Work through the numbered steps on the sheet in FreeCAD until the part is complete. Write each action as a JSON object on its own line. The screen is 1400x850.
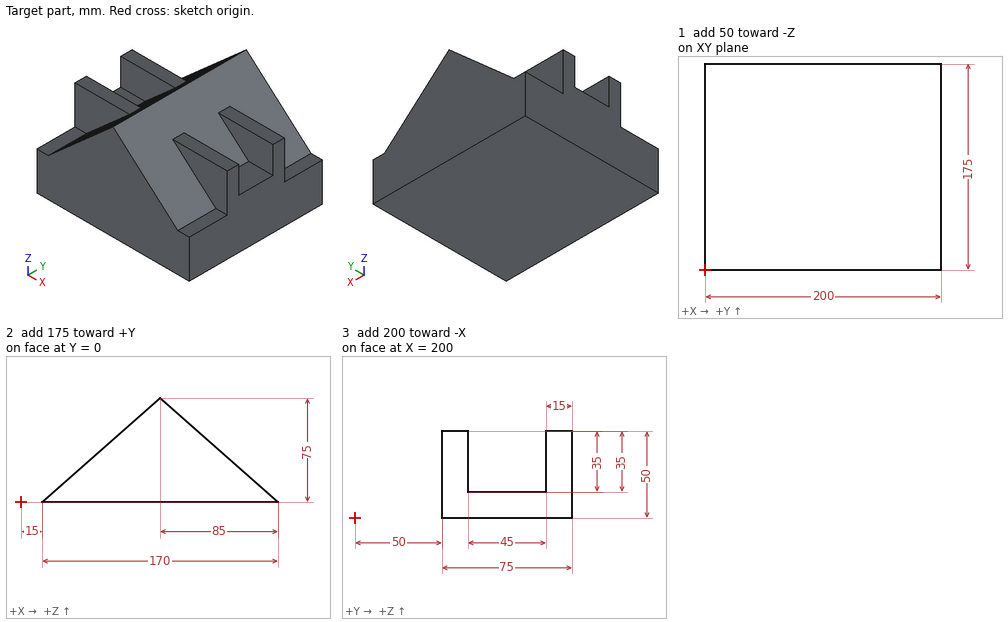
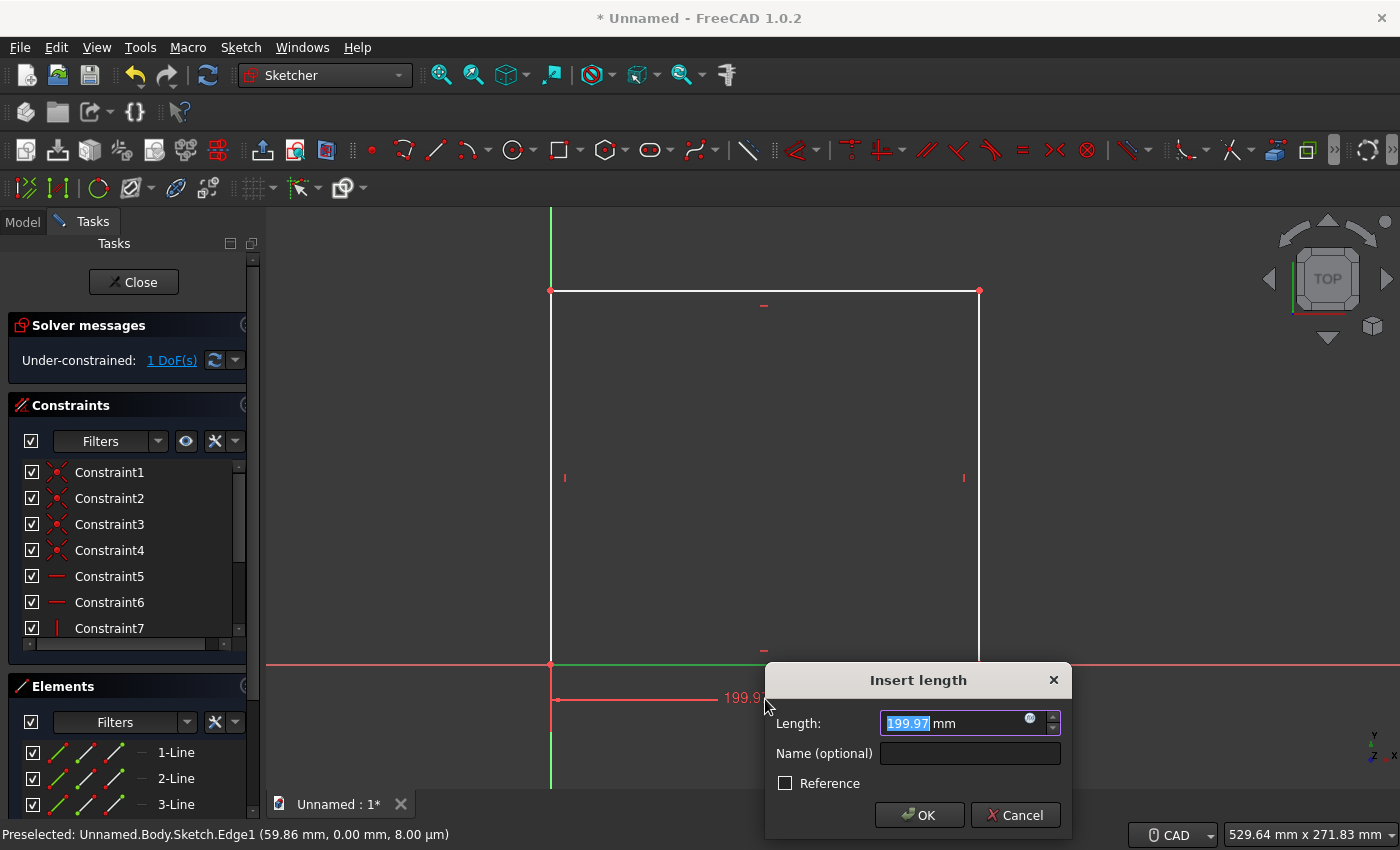
{"action": "type", "text": "200"}
{"action": "key", "text": "Return"}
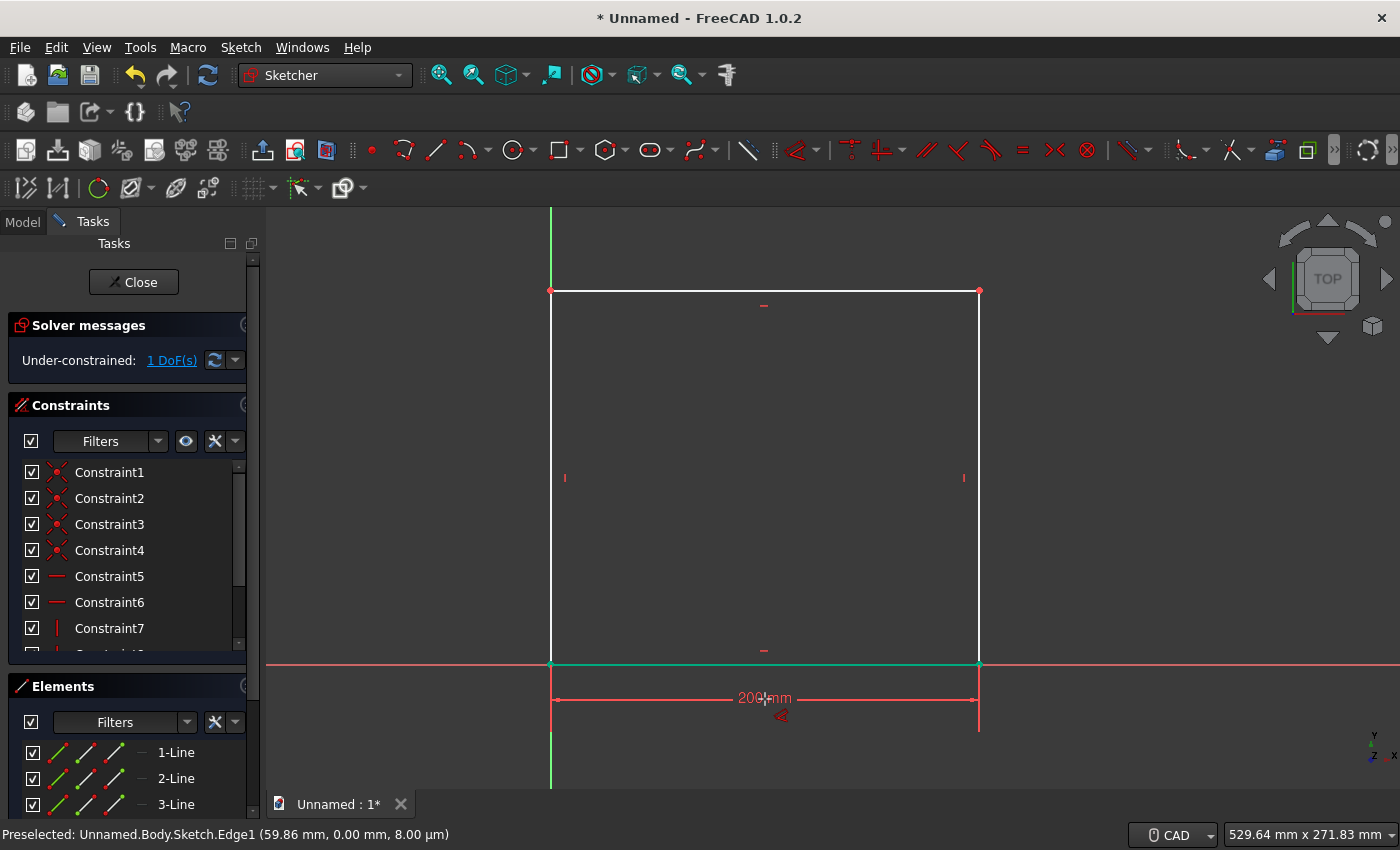
{"action": "left_click", "coordinate": [979, 553]}
{"action": "left_click", "coordinate": [1013, 478]}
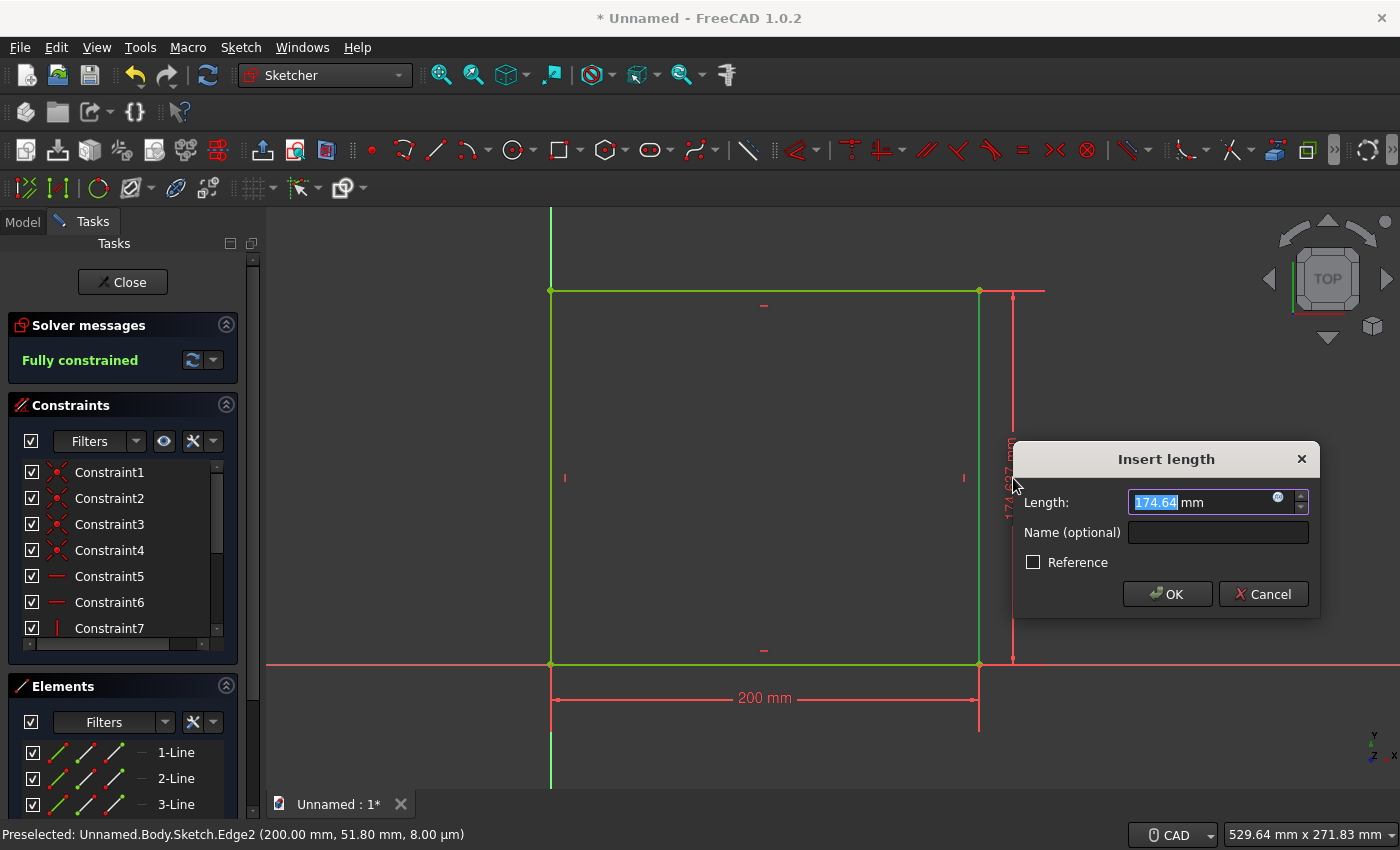
{"action": "type", "text": "175"}
{"action": "key", "text": "Return"}
{"action": "key", "text": "Escape"}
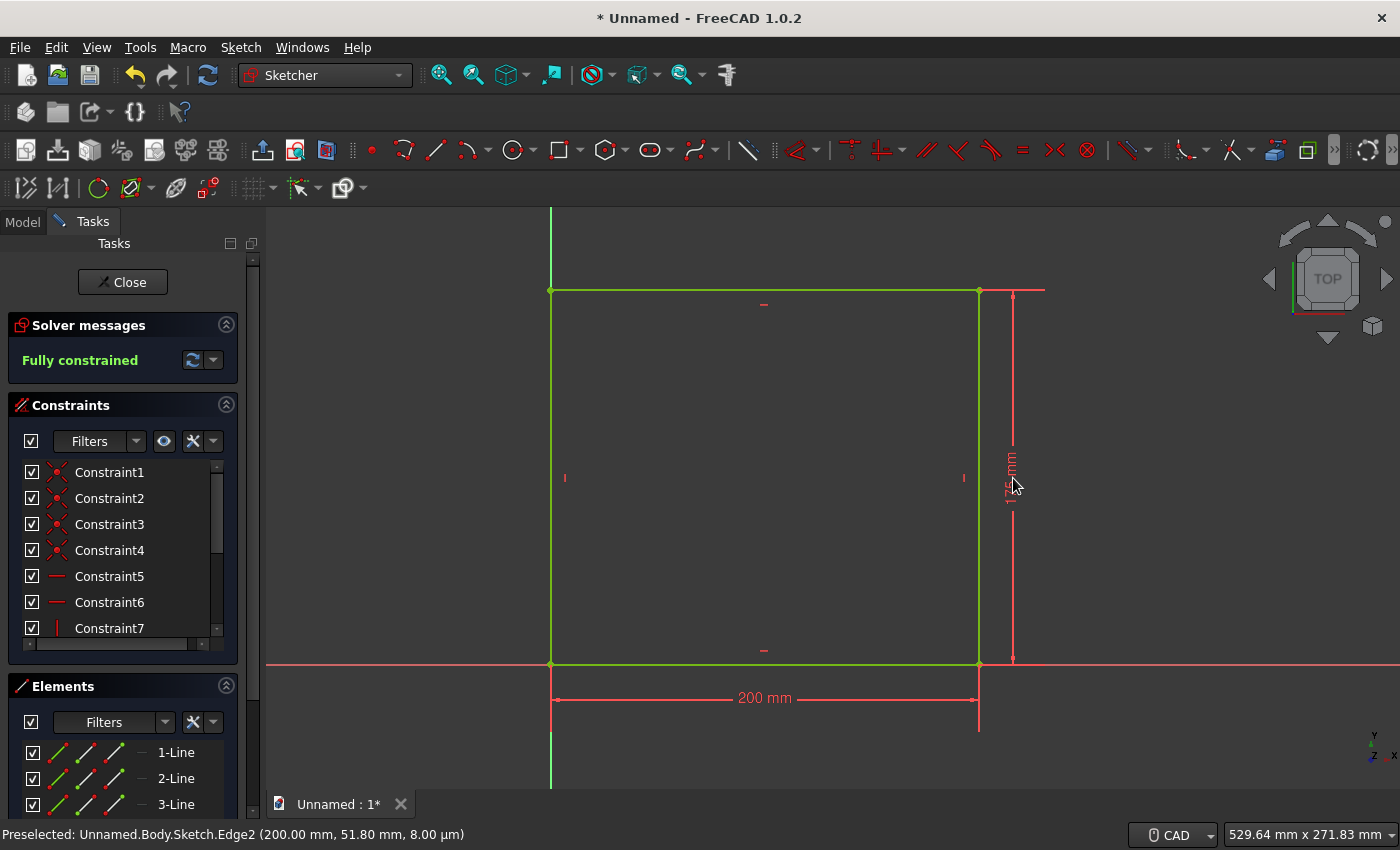
{"action": "left_click", "coordinate": [123, 282]}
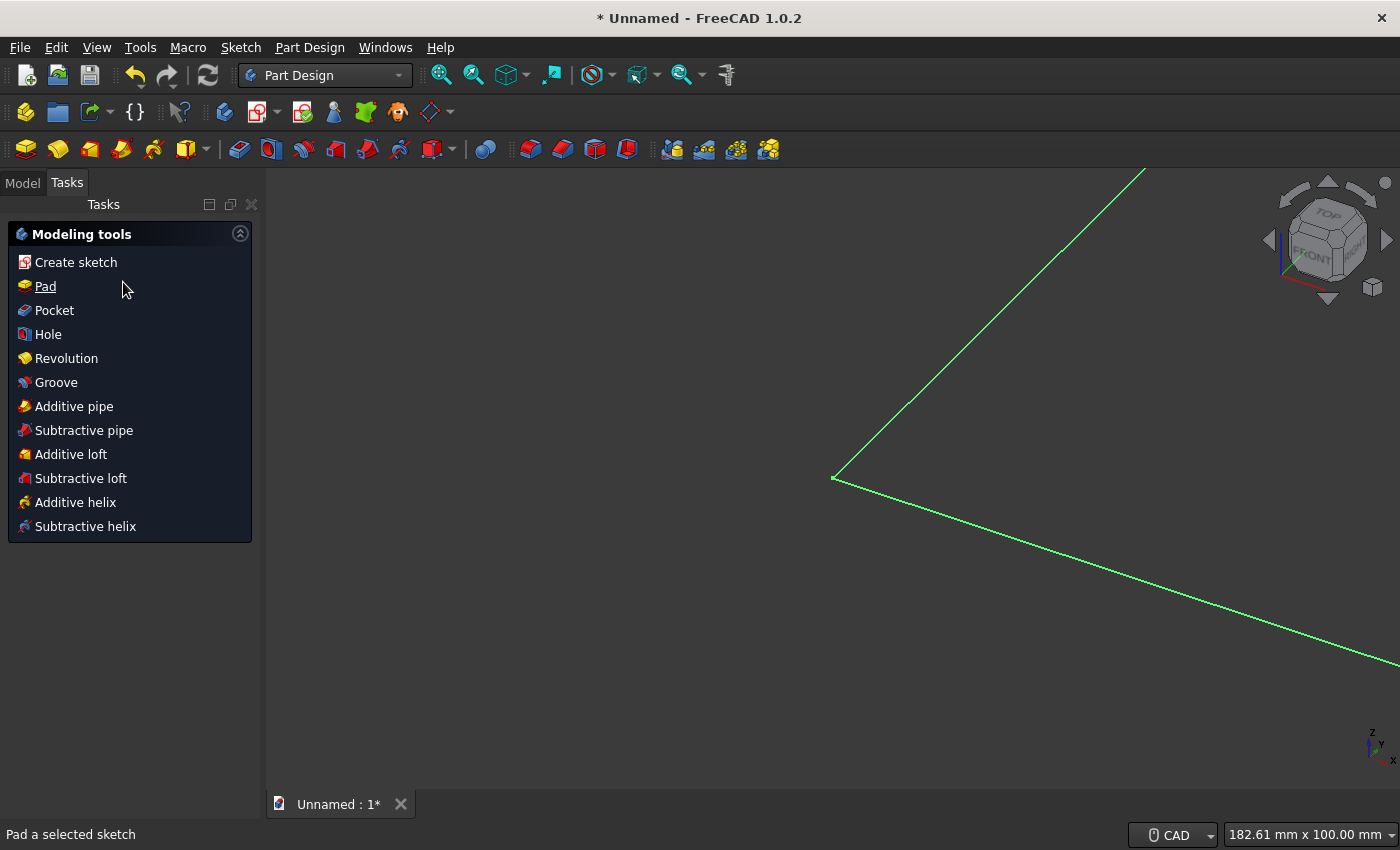
{"action": "left_click", "coordinate": [26, 150]}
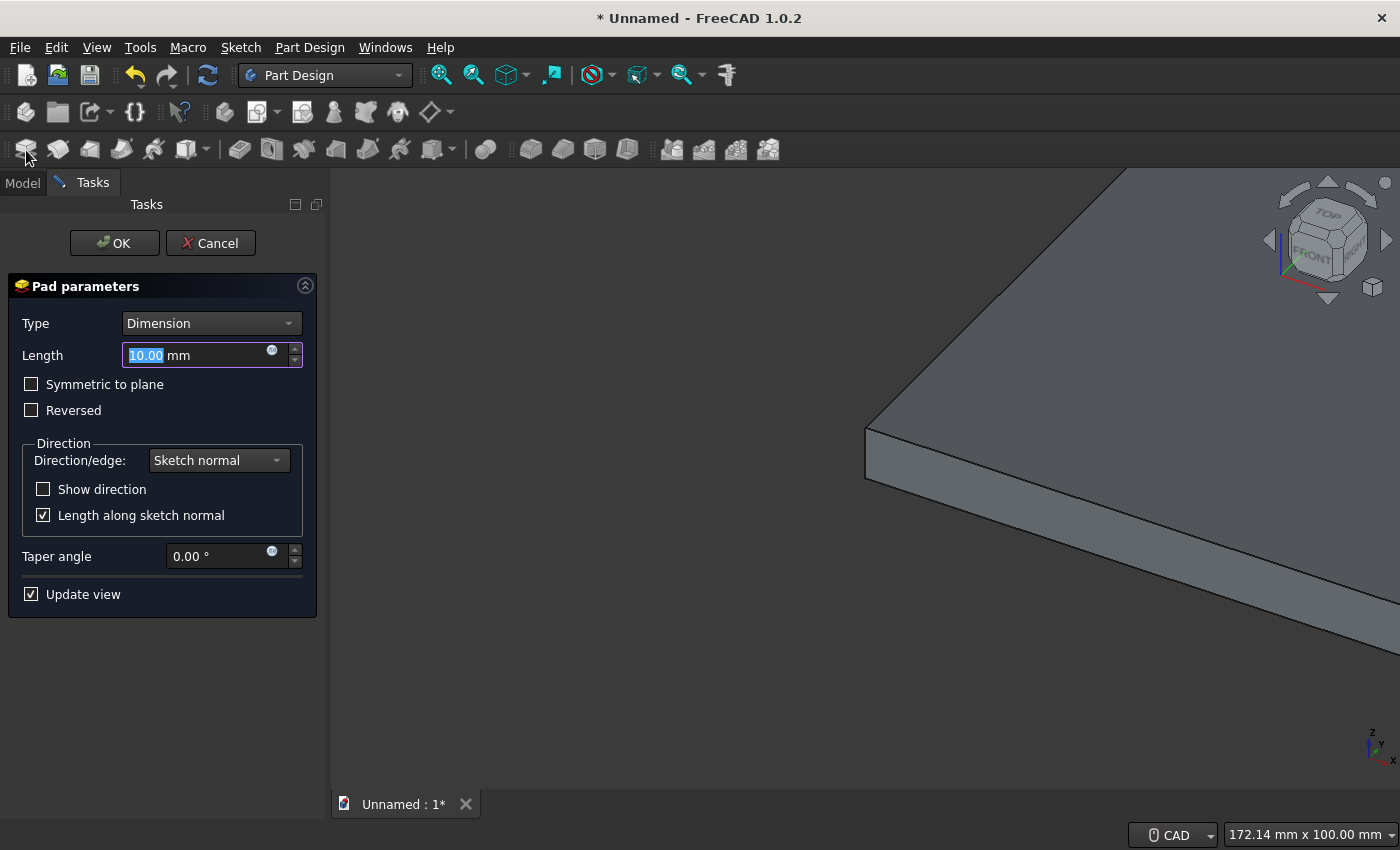
{"action": "type", "text": "50"}
{"action": "key", "text": "Tab"}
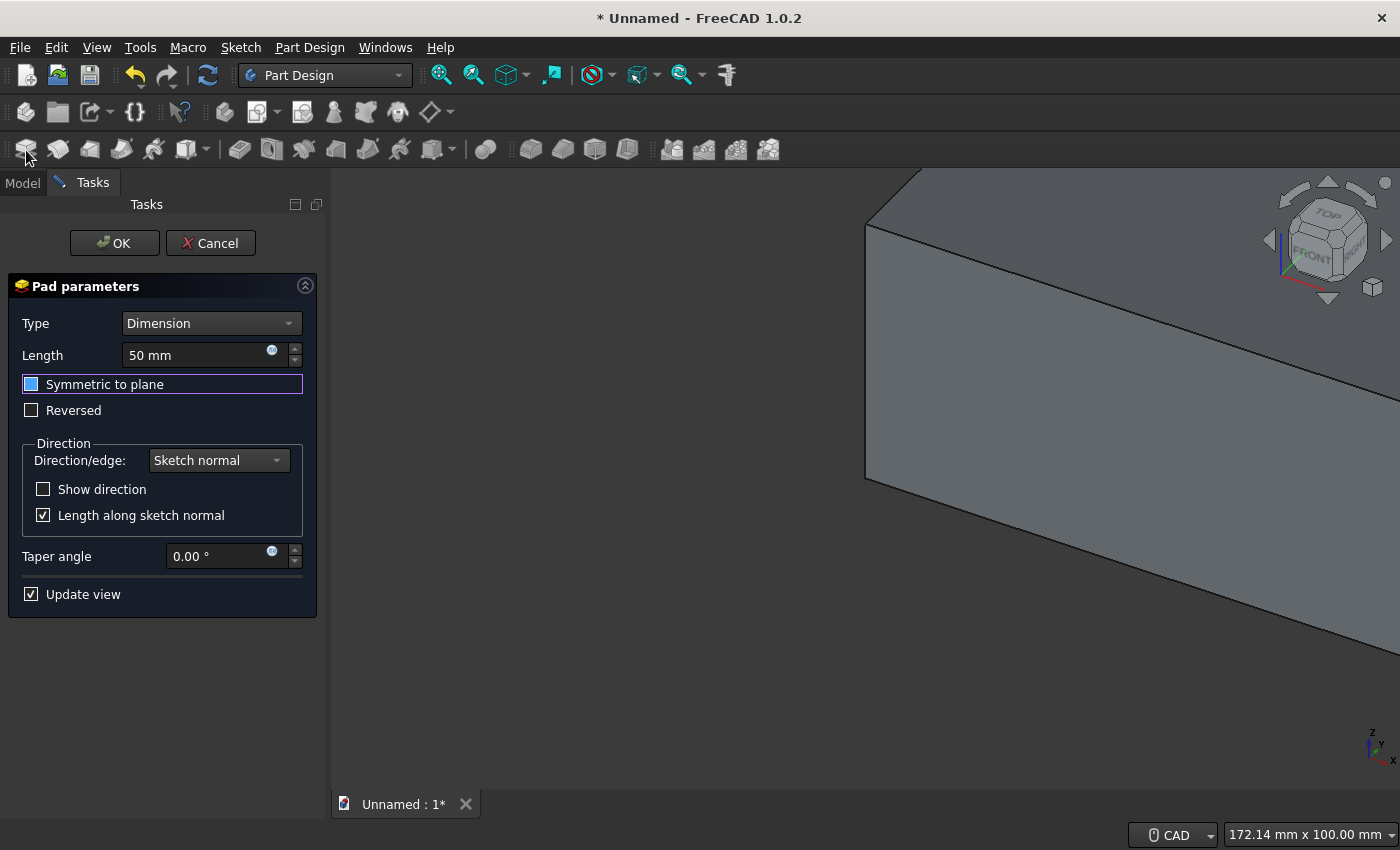
{"action": "left_click", "coordinate": [30, 410]}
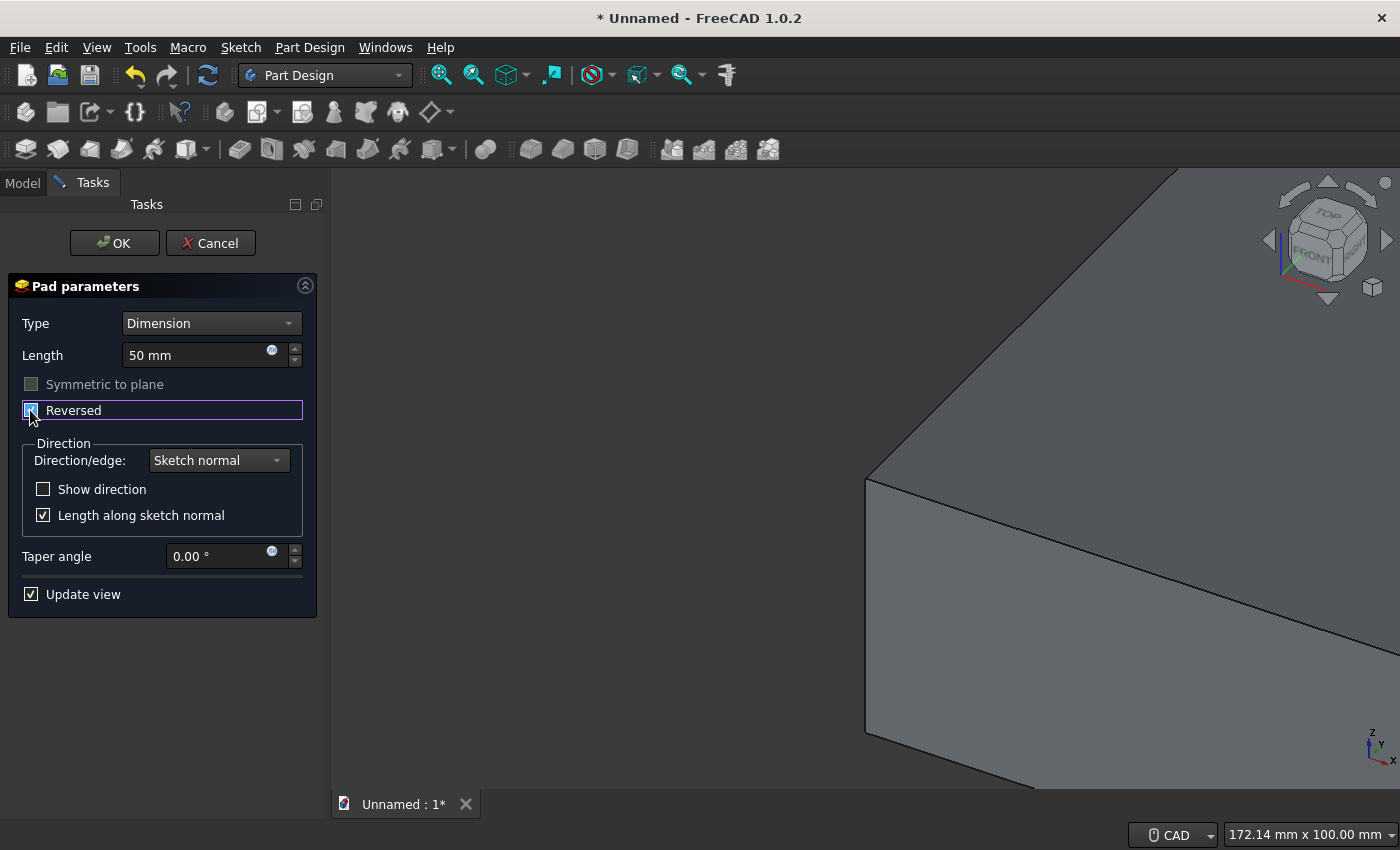
{"action": "left_click", "coordinate": [115, 243]}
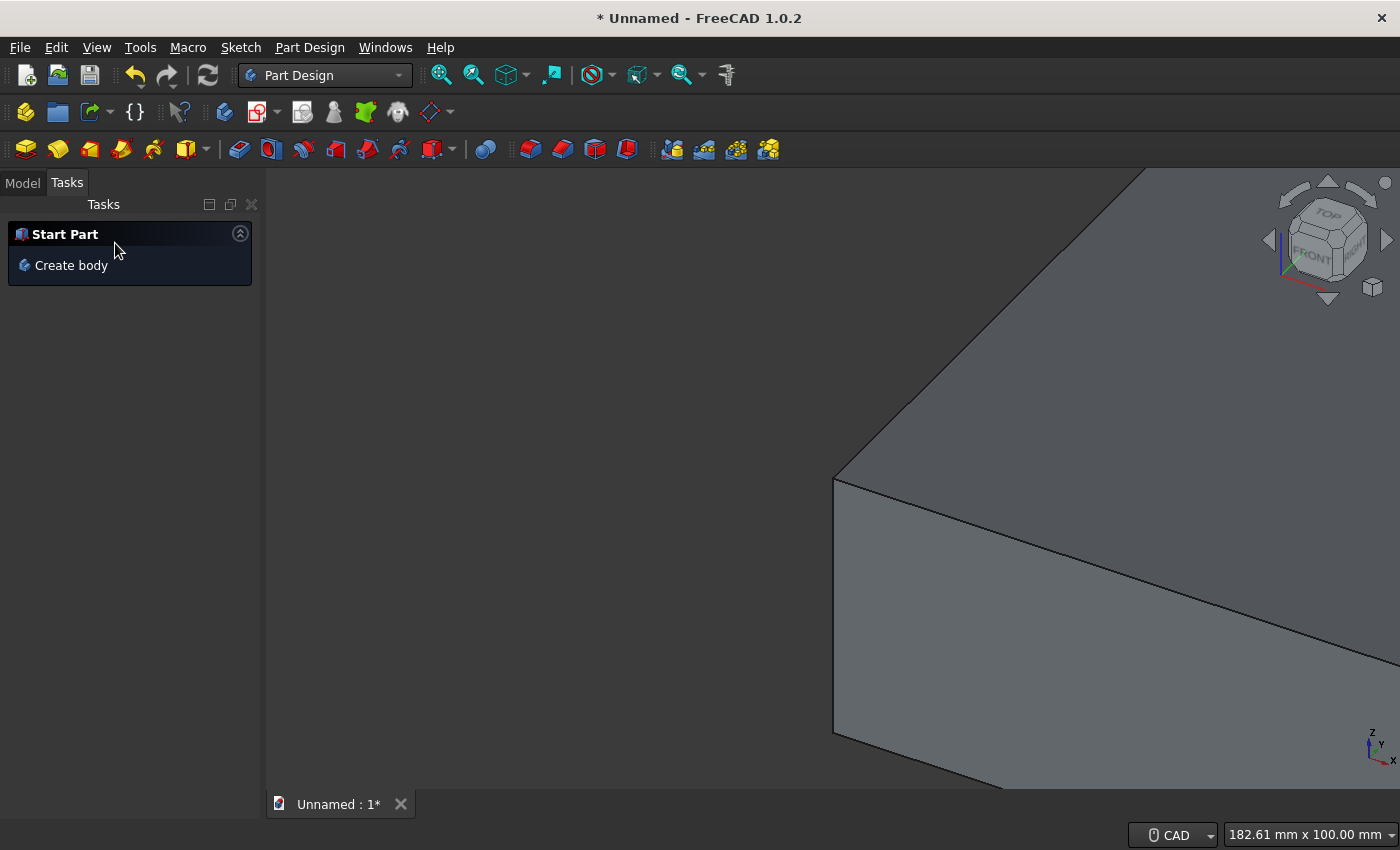
{"action": "left_click", "coordinate": [442, 76]}